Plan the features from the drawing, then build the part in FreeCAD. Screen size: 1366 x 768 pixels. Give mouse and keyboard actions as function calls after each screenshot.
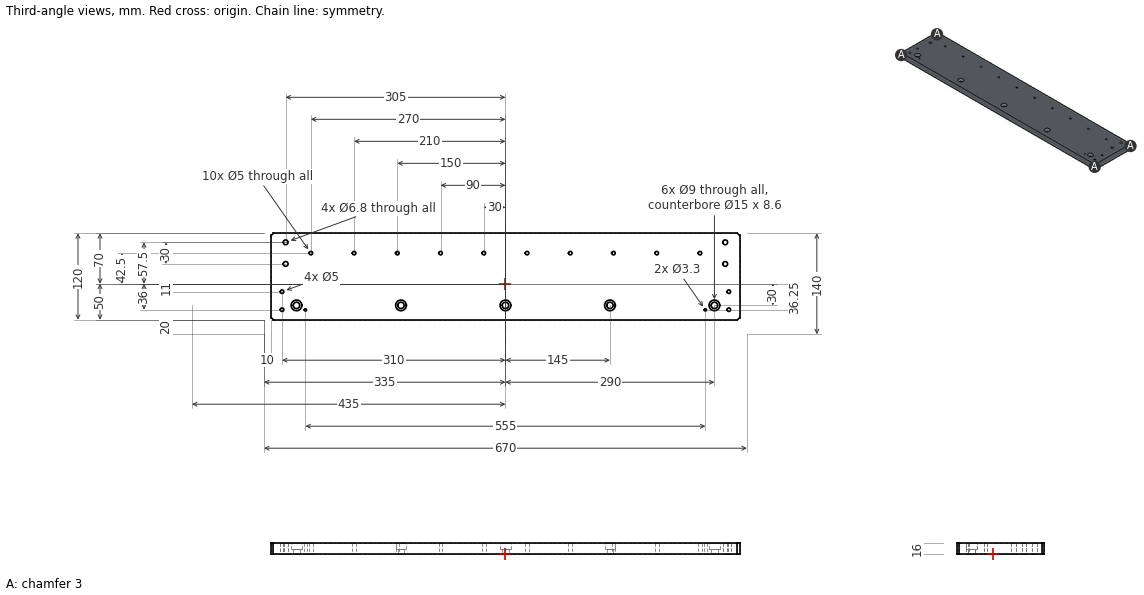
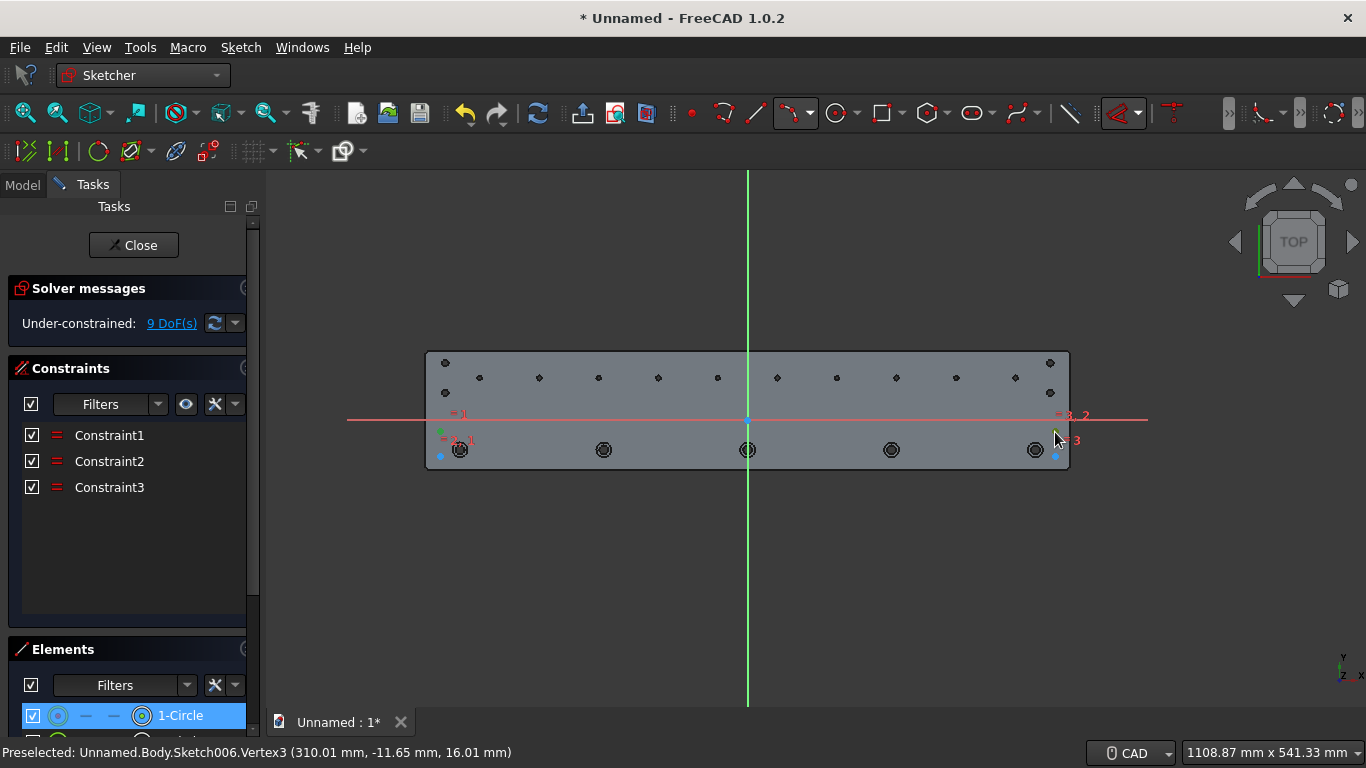
click(748, 645)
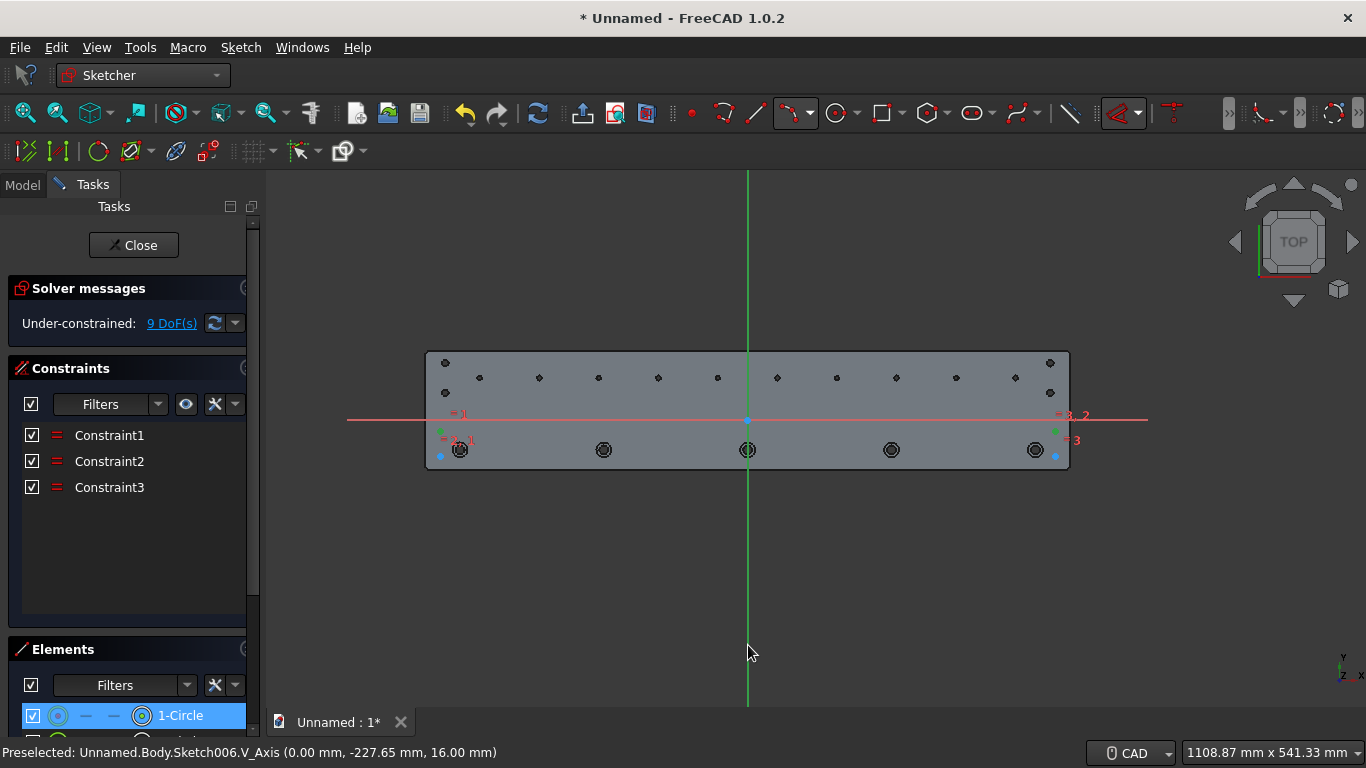
key(s)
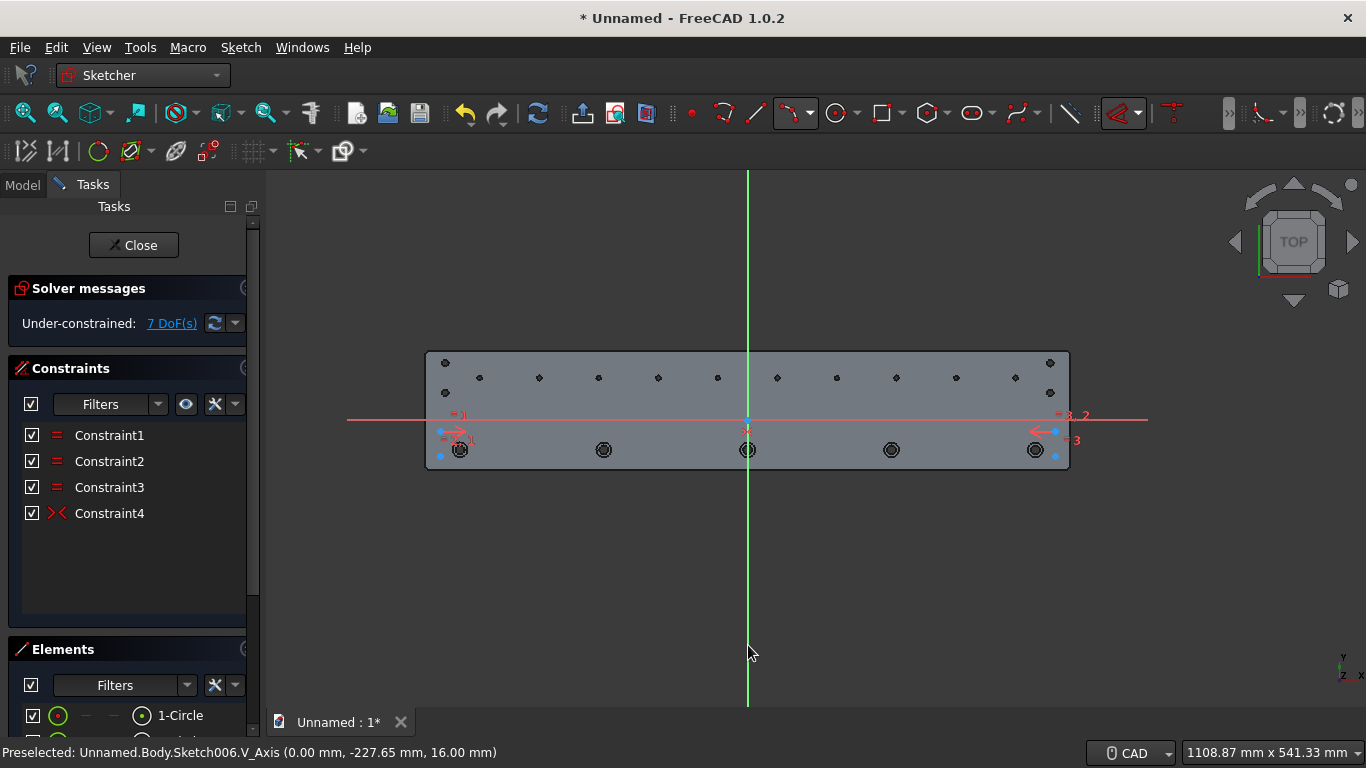
click(440, 457)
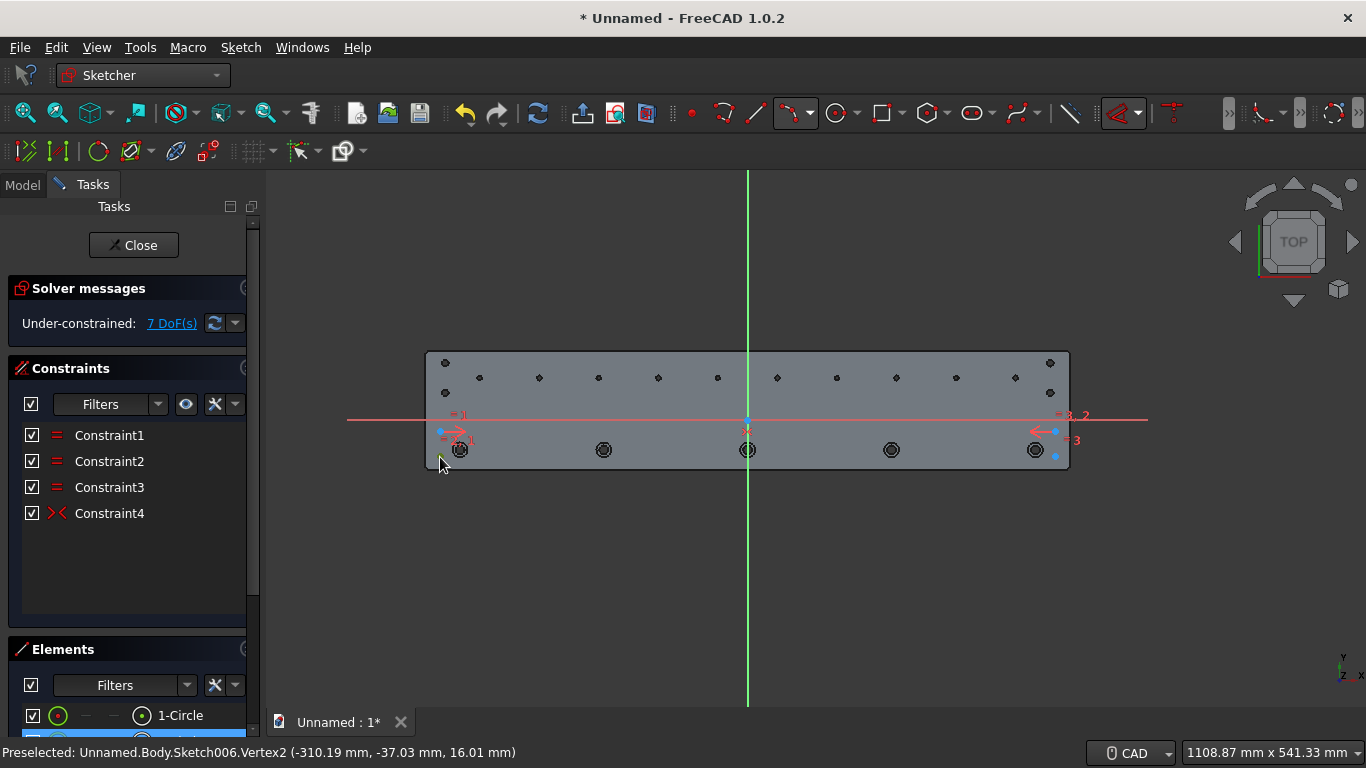
click(1055, 457)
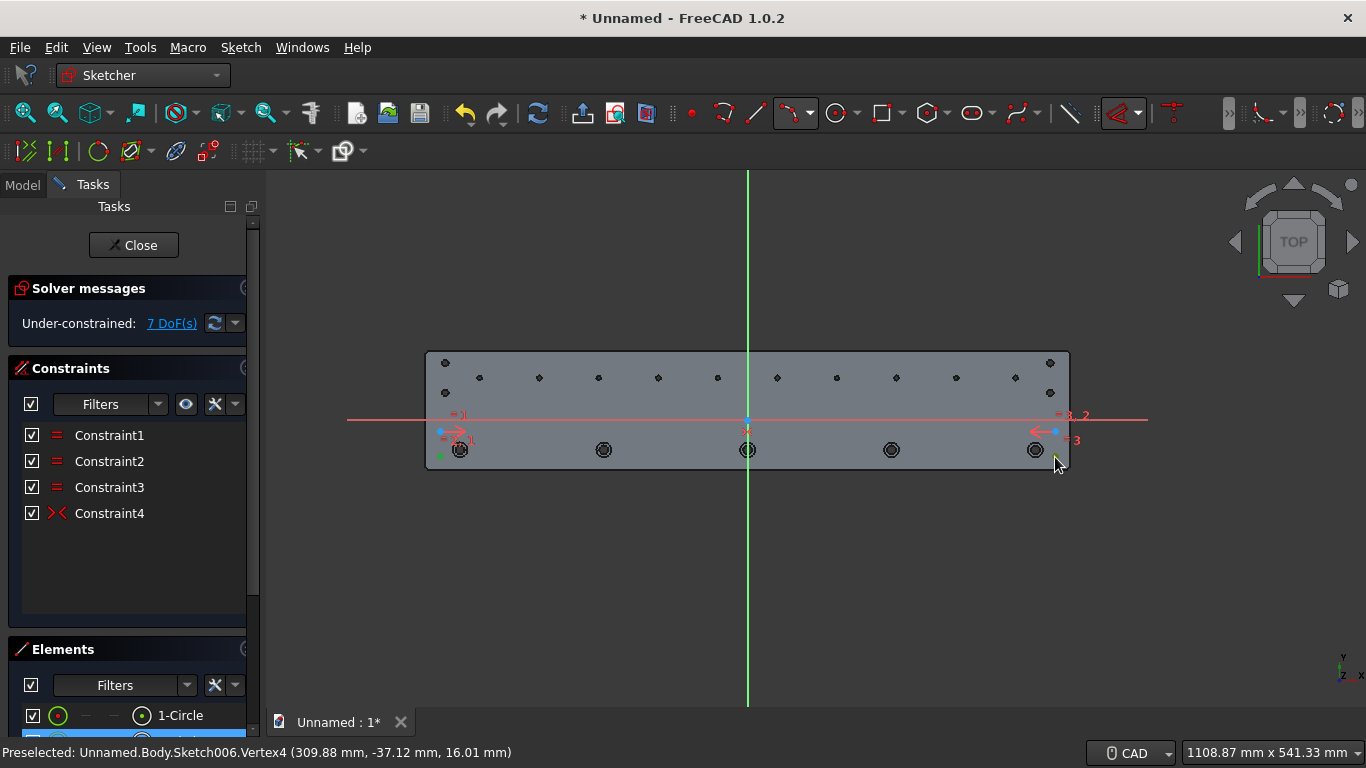
click(748, 645)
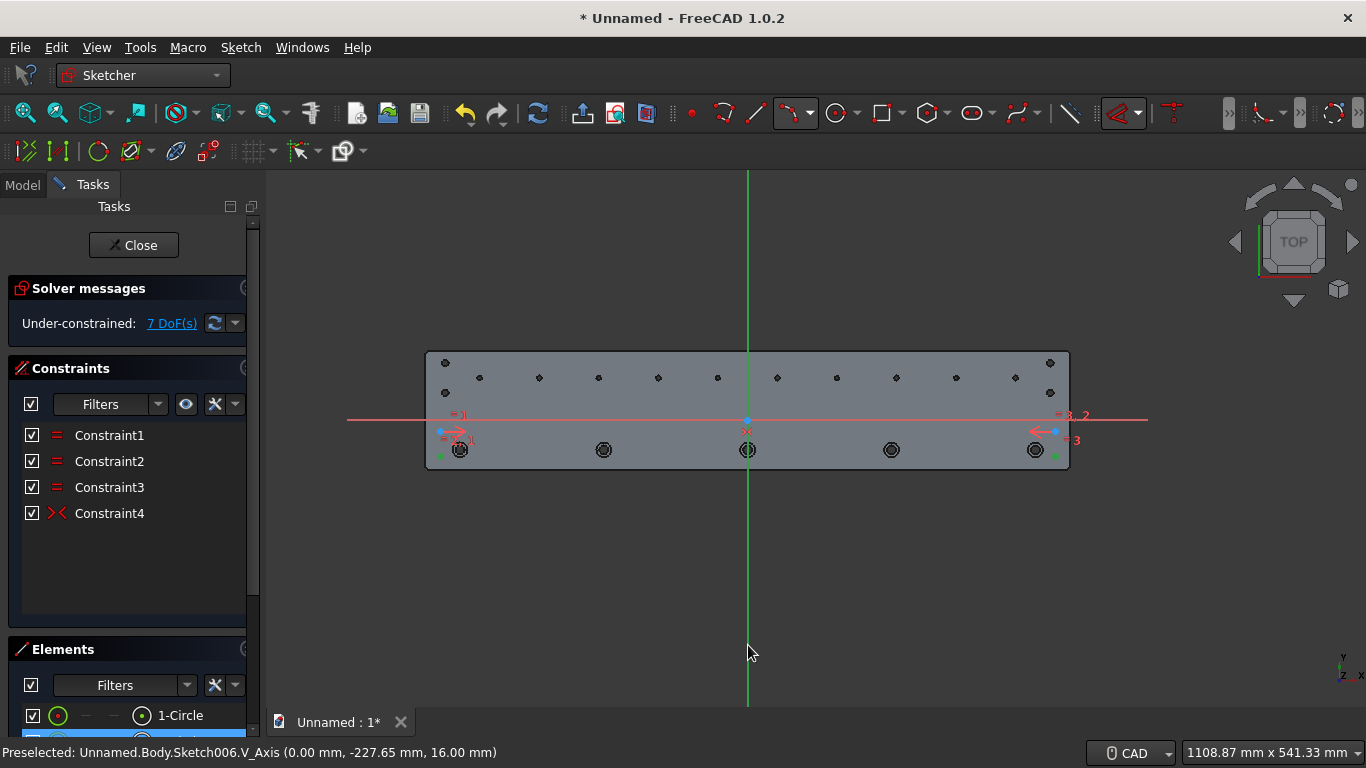
key(s)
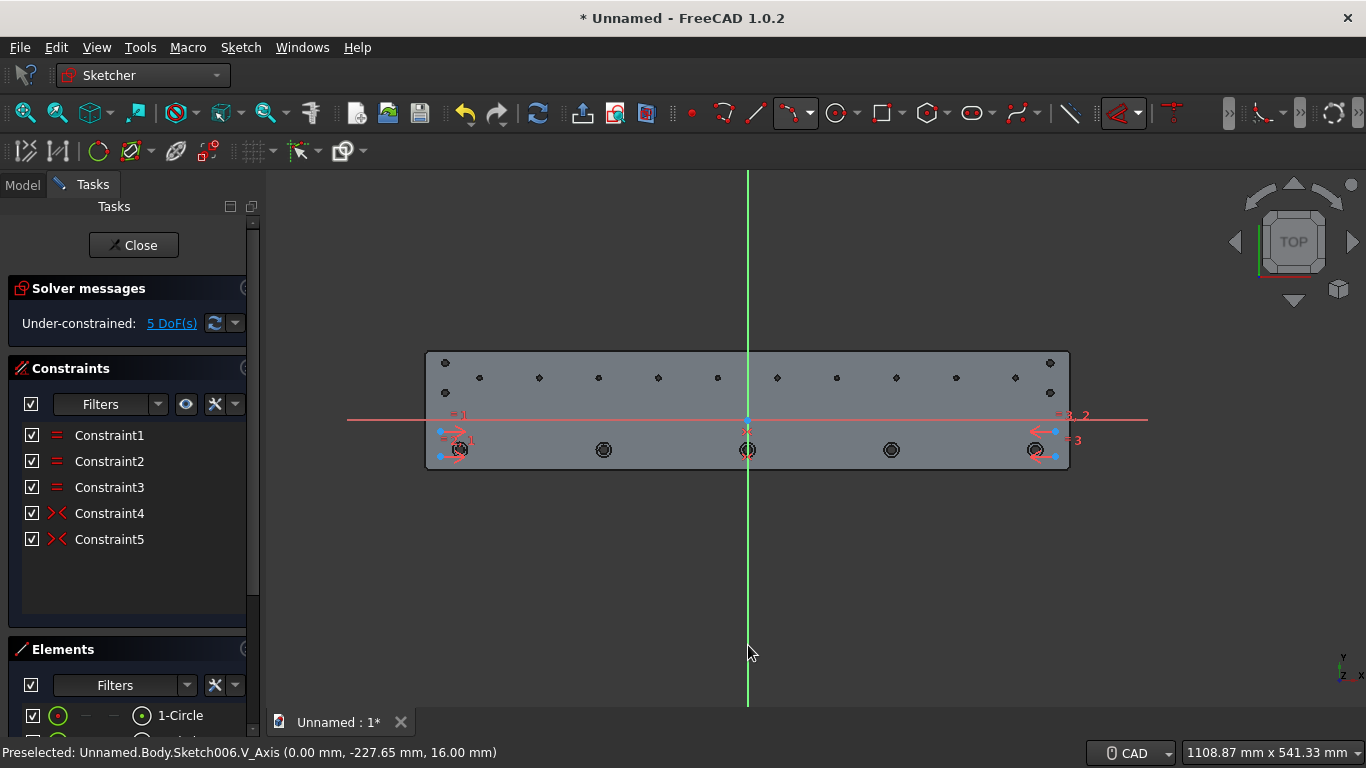
scroll(442, 430, up, 11)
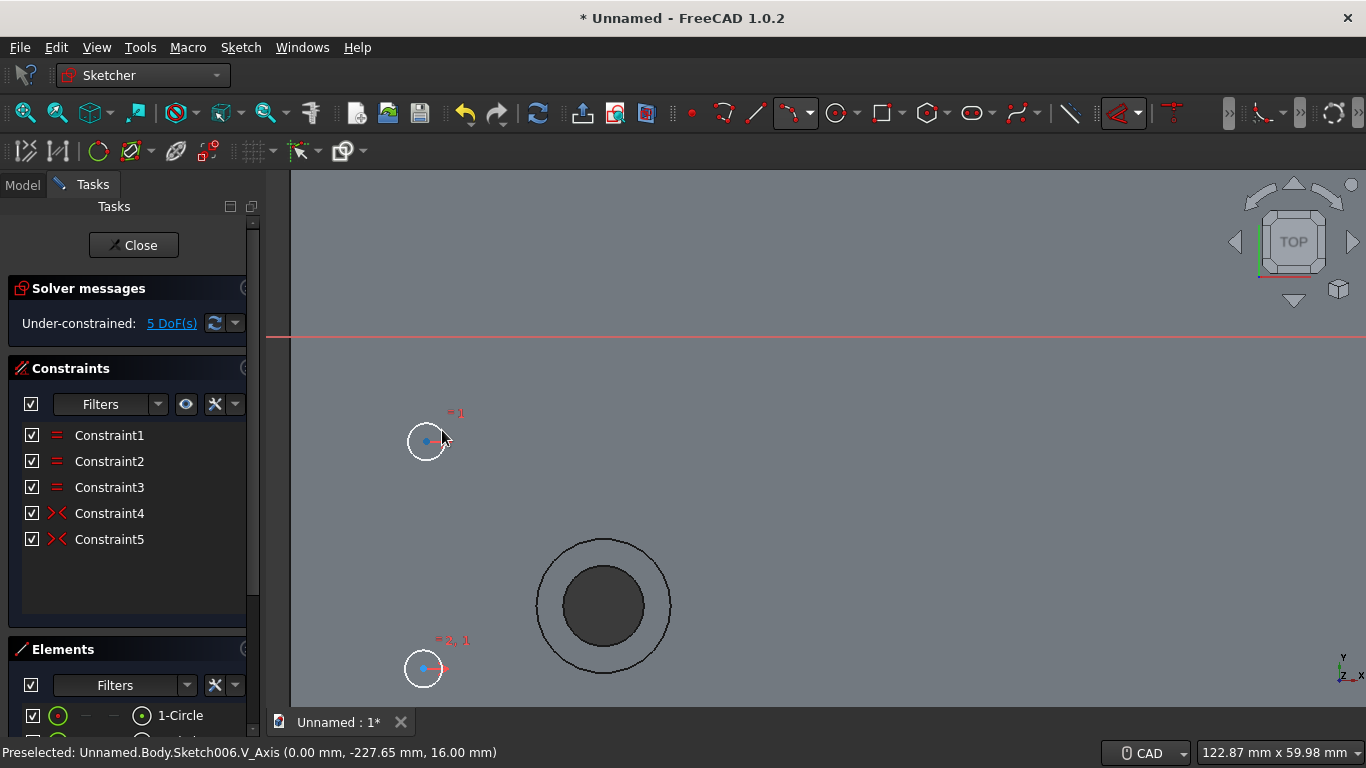
click(439, 429)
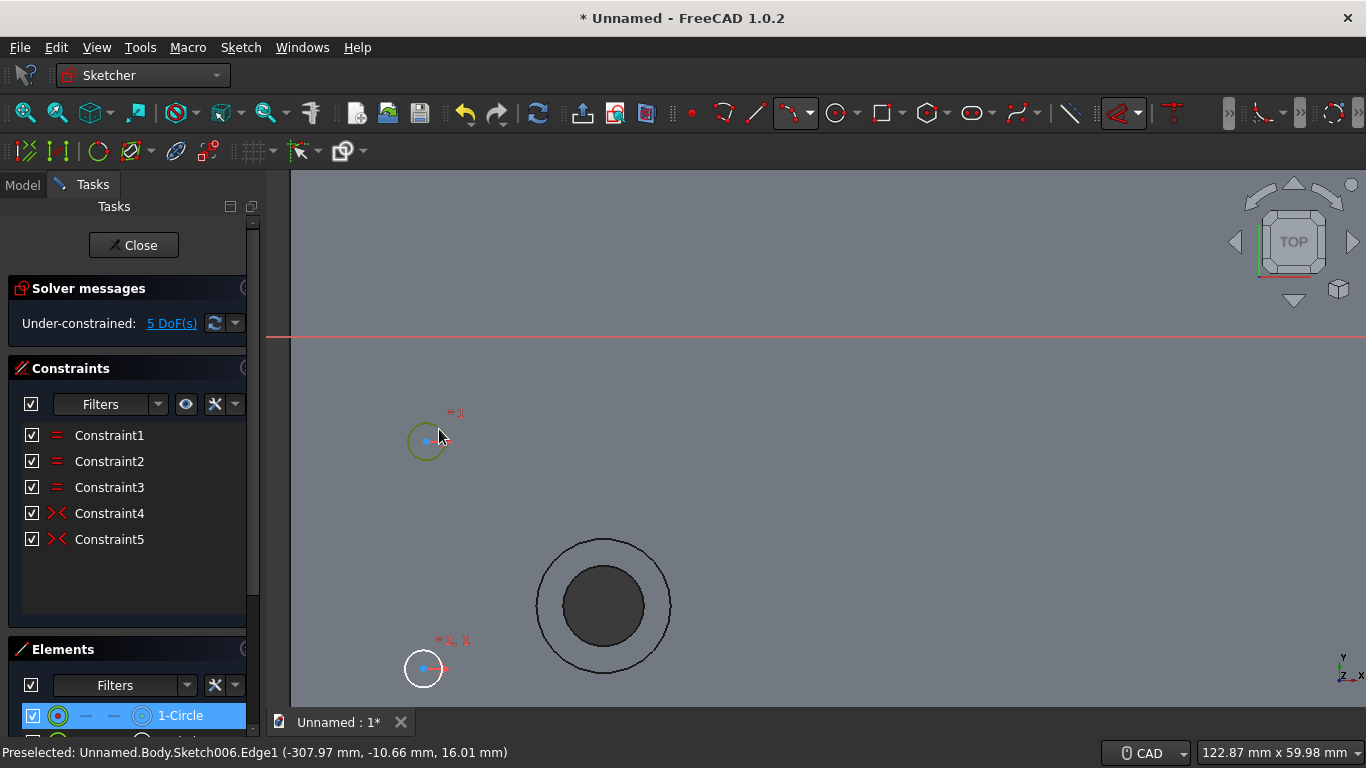
click(1140, 114)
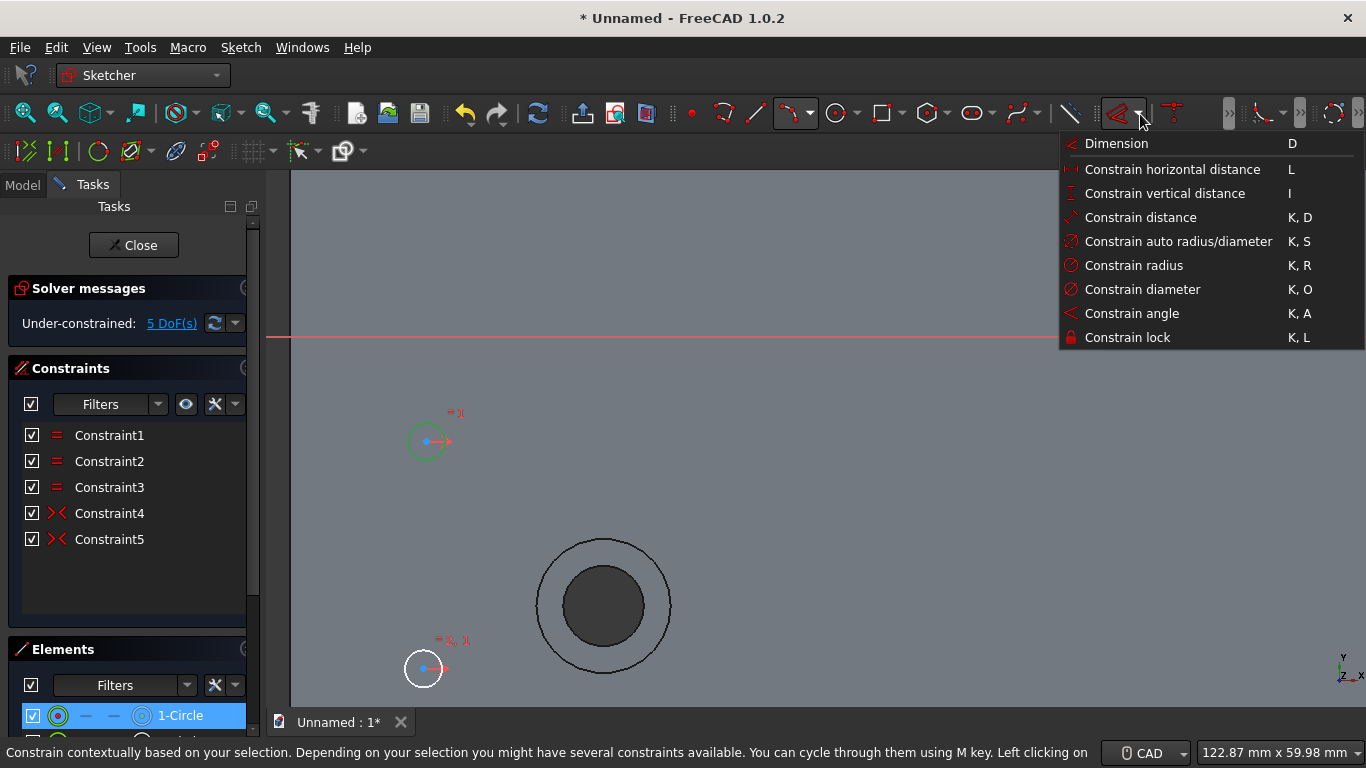
click(1212, 289)